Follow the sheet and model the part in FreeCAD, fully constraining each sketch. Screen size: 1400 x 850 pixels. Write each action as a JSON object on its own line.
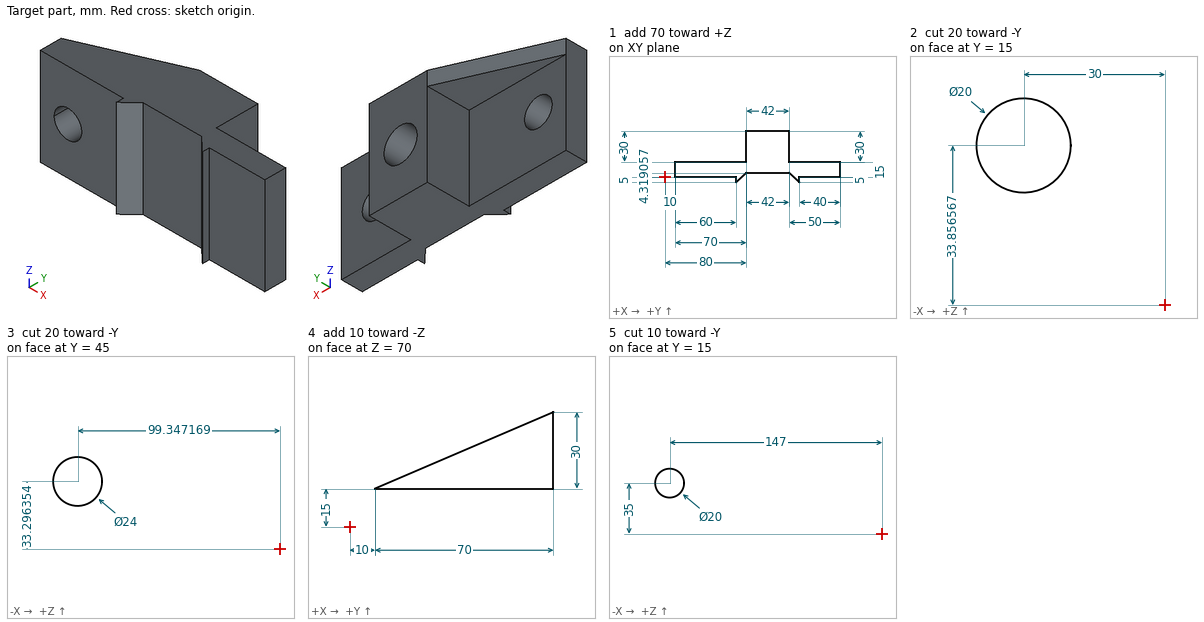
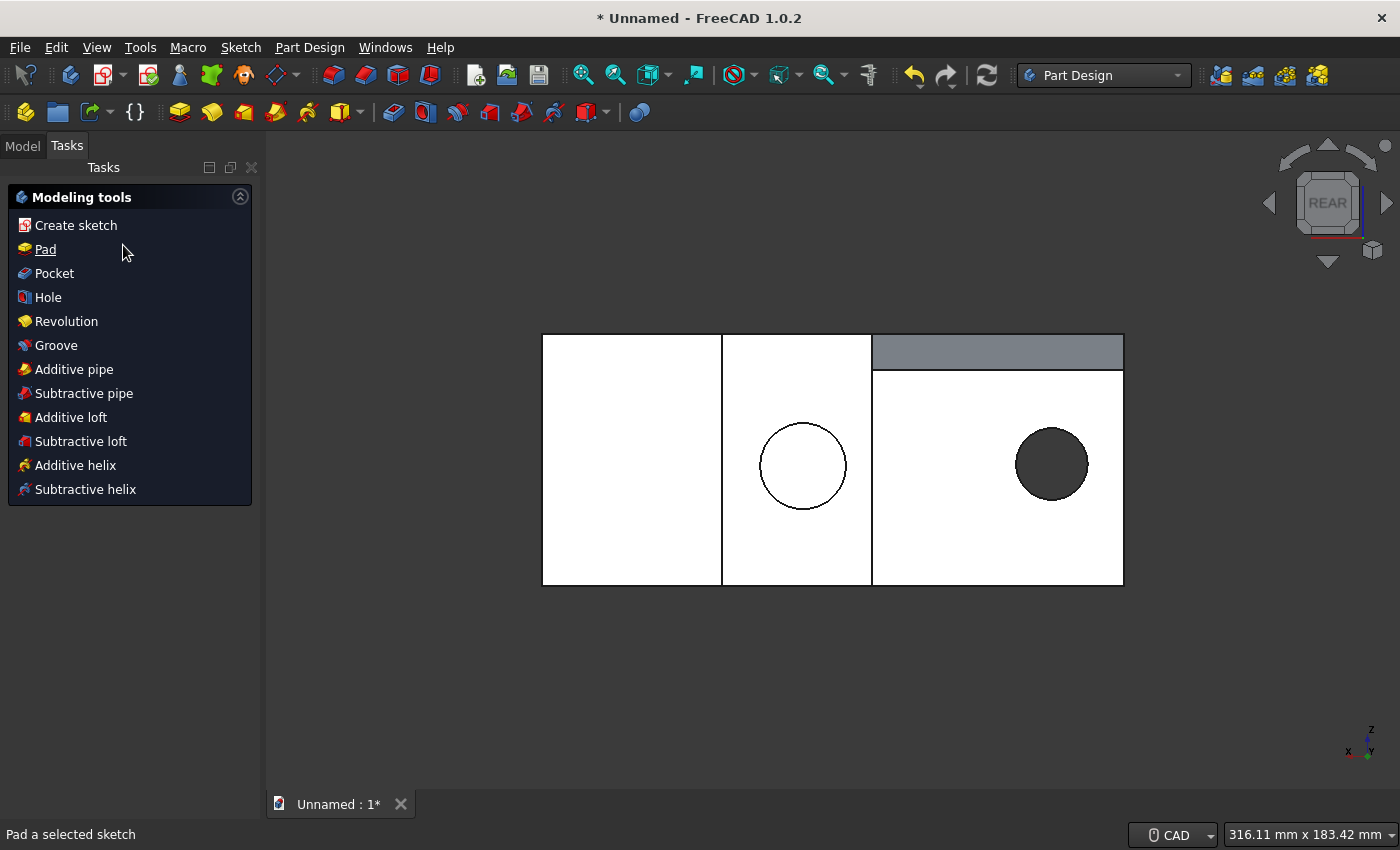
{"action": "left_click", "coordinate": [394, 112]}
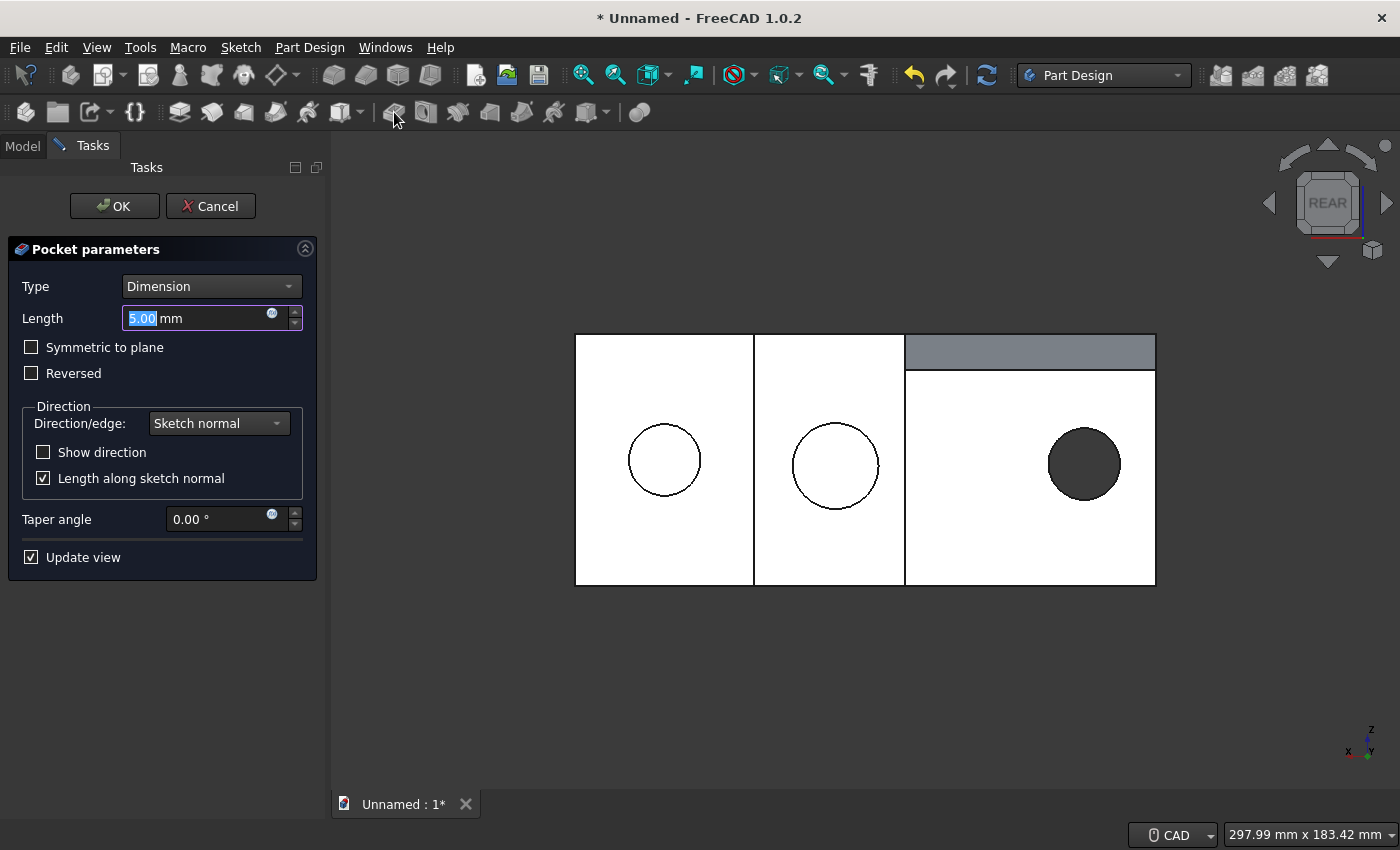
{"action": "type", "text": "10"}
{"action": "key", "text": "Tab"}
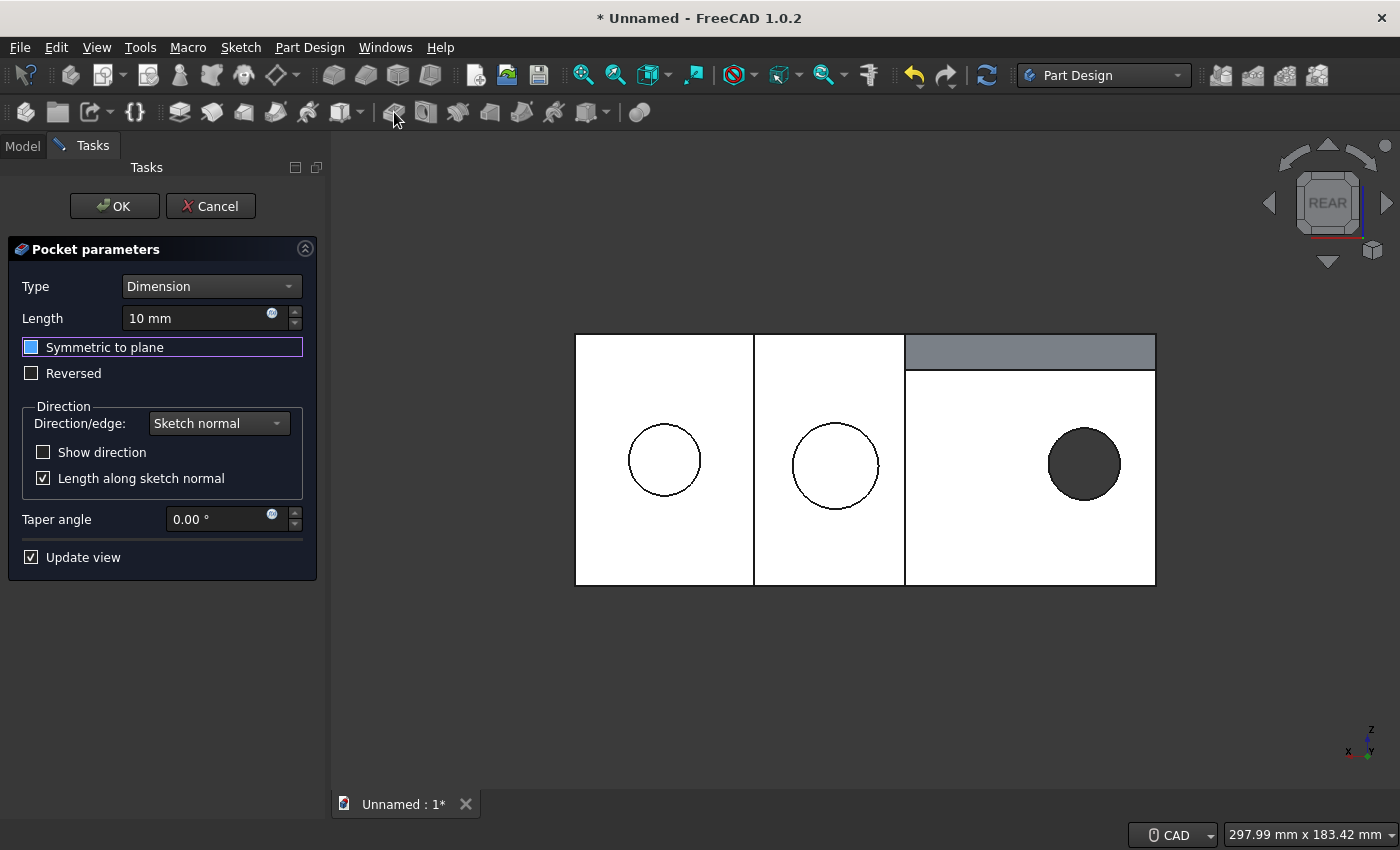
{"action": "left_click", "coordinate": [115, 206]}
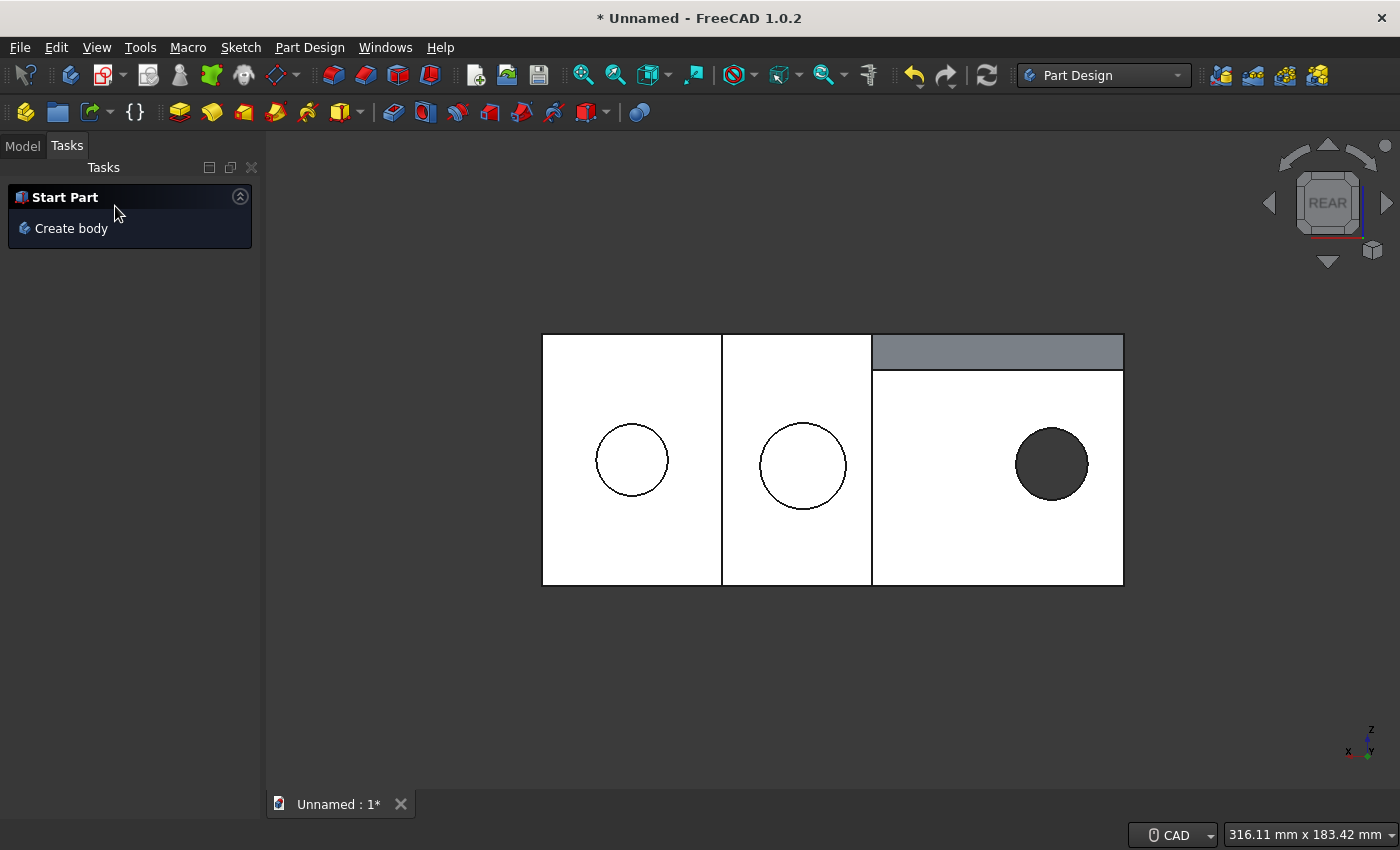
{"action": "key", "text": "0"}